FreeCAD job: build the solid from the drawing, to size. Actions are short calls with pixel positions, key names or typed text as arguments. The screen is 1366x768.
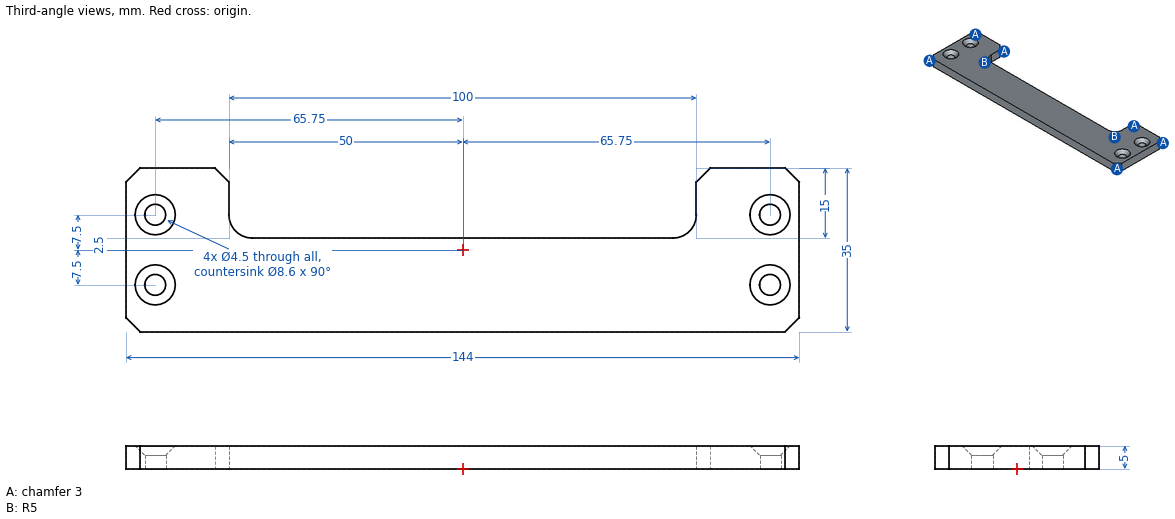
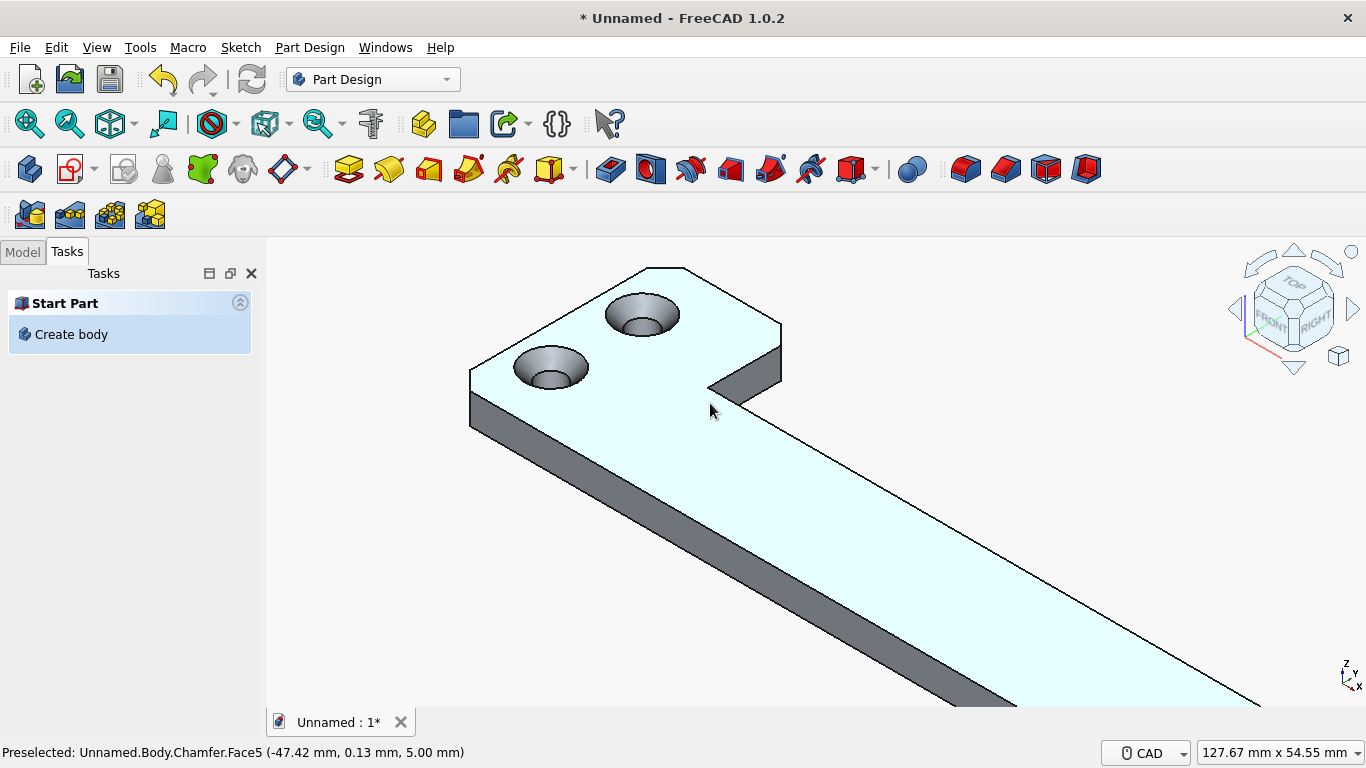
key(v)
key(f)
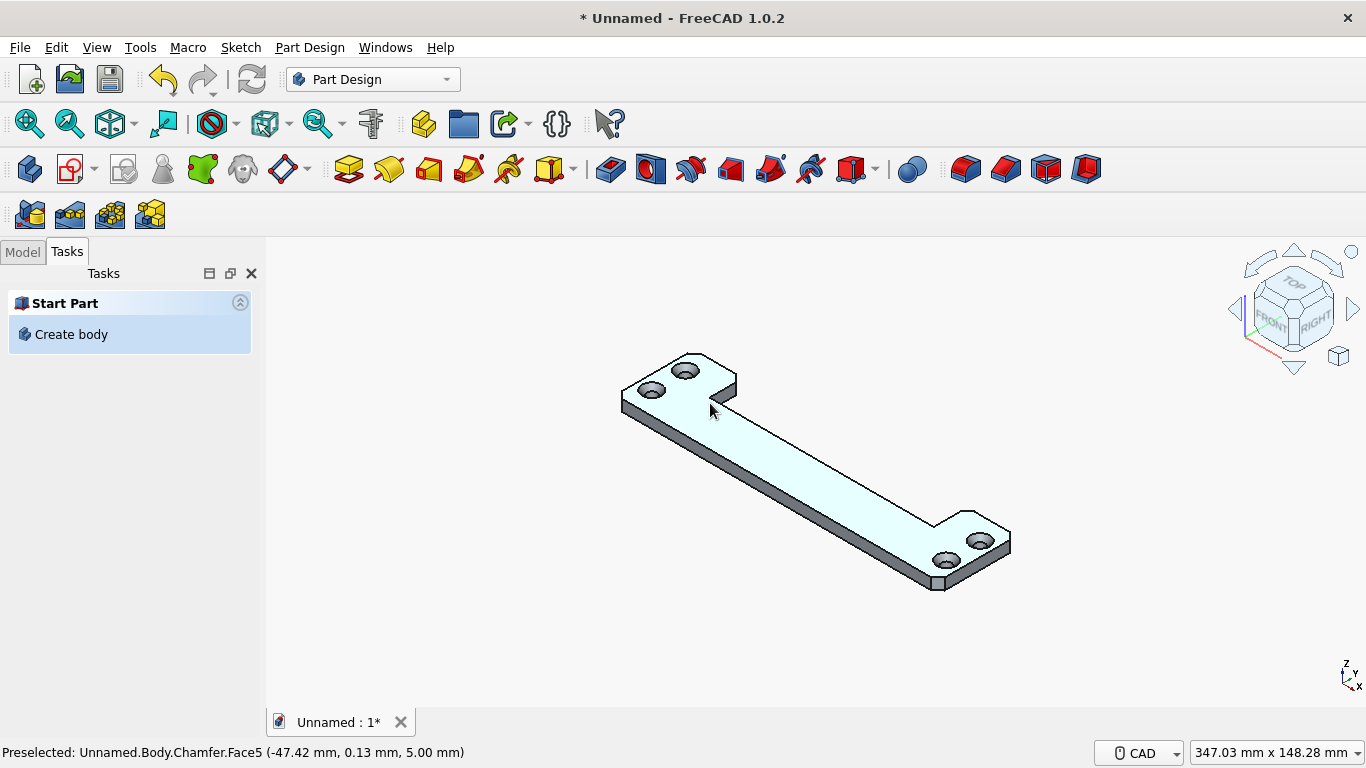
key(2)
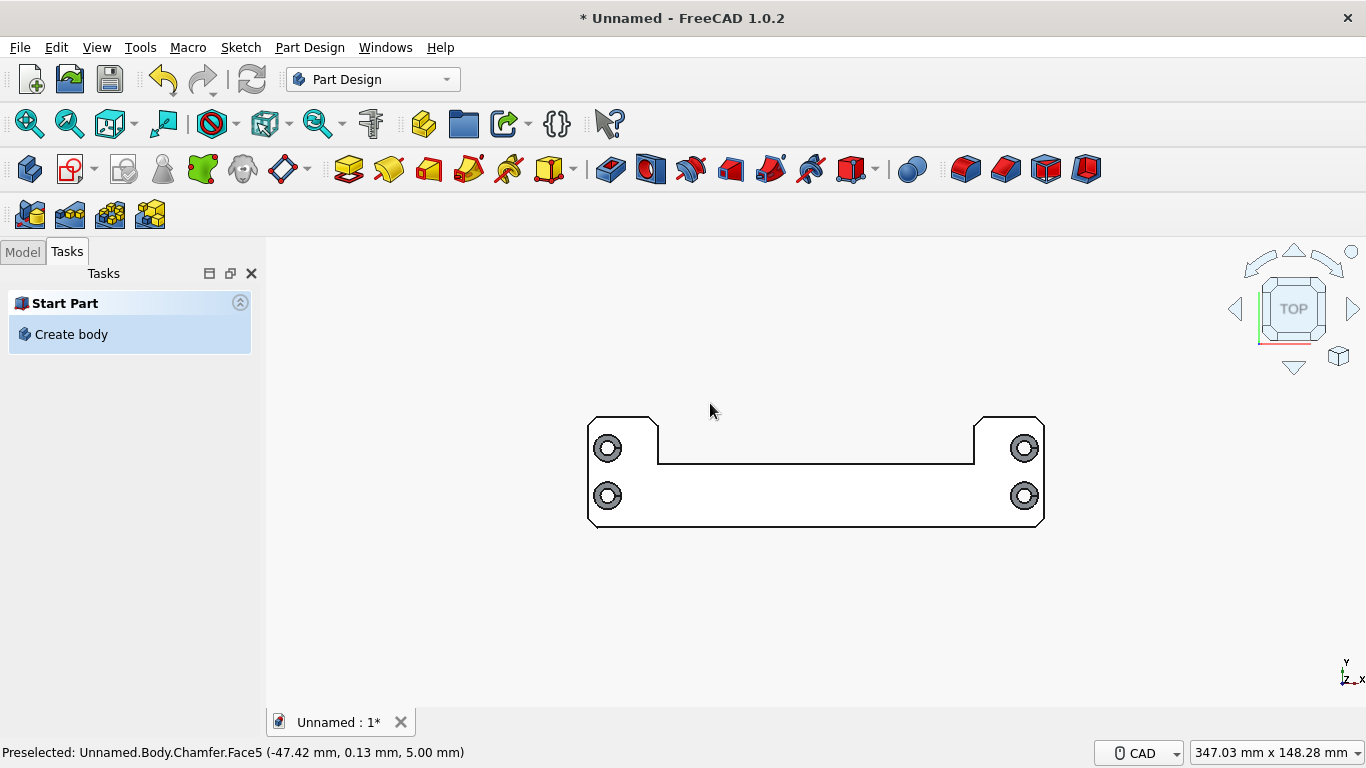
key(v)
key(f)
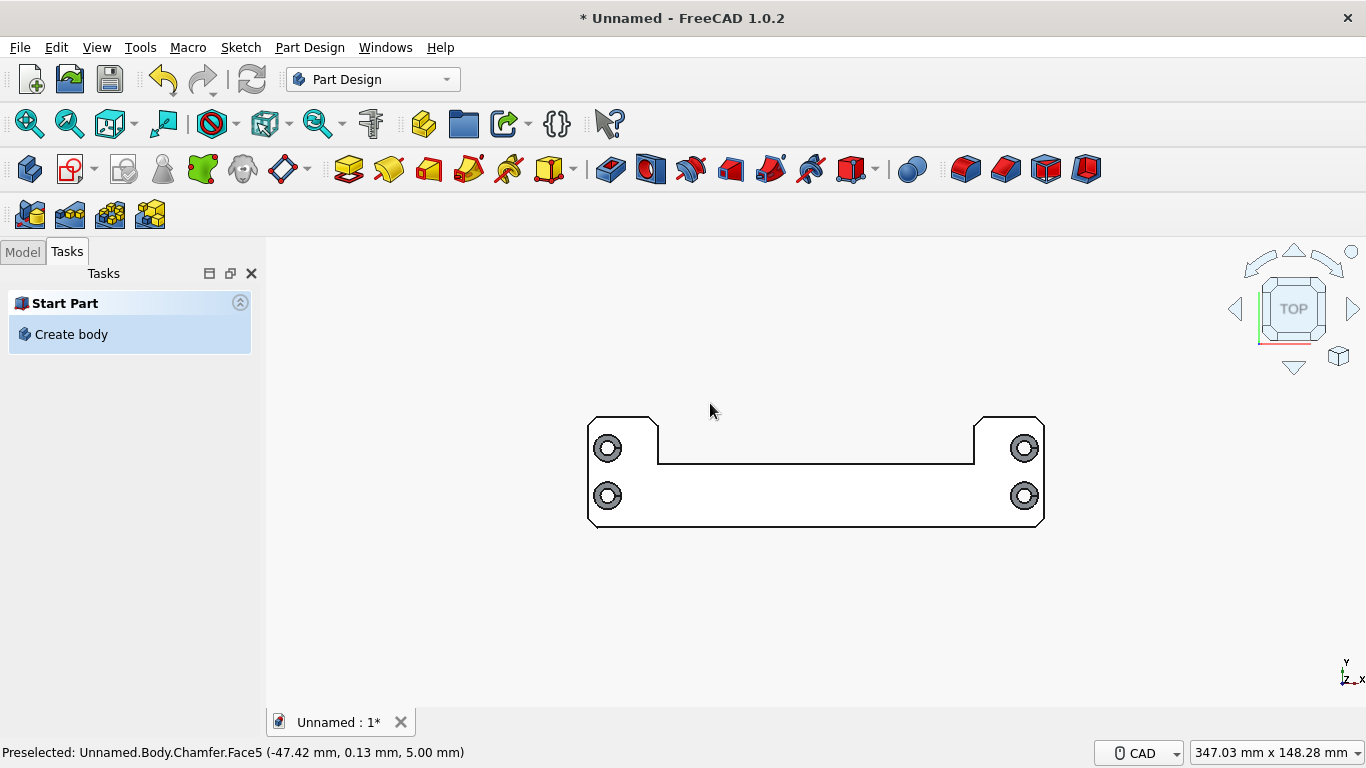
scroll(658, 463, up, 5)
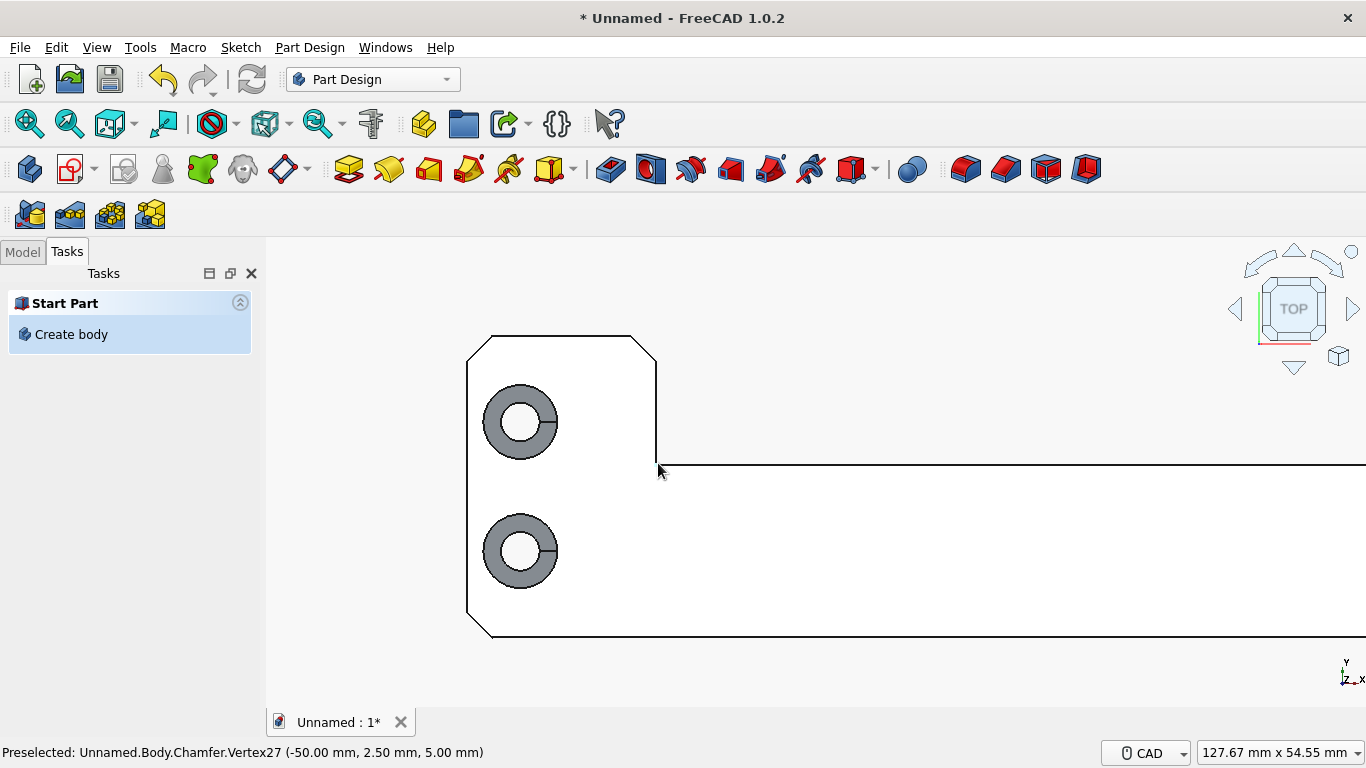
key(v)
key(f)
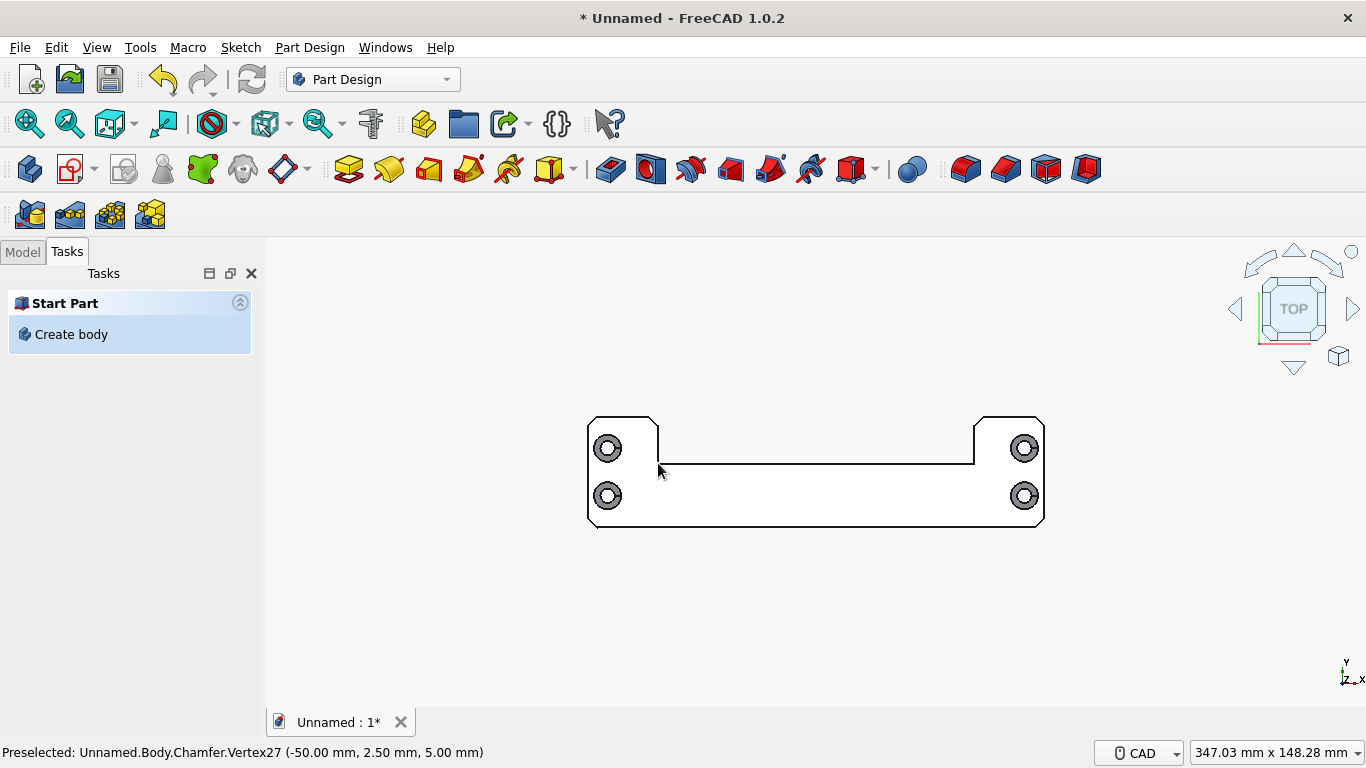
key(1)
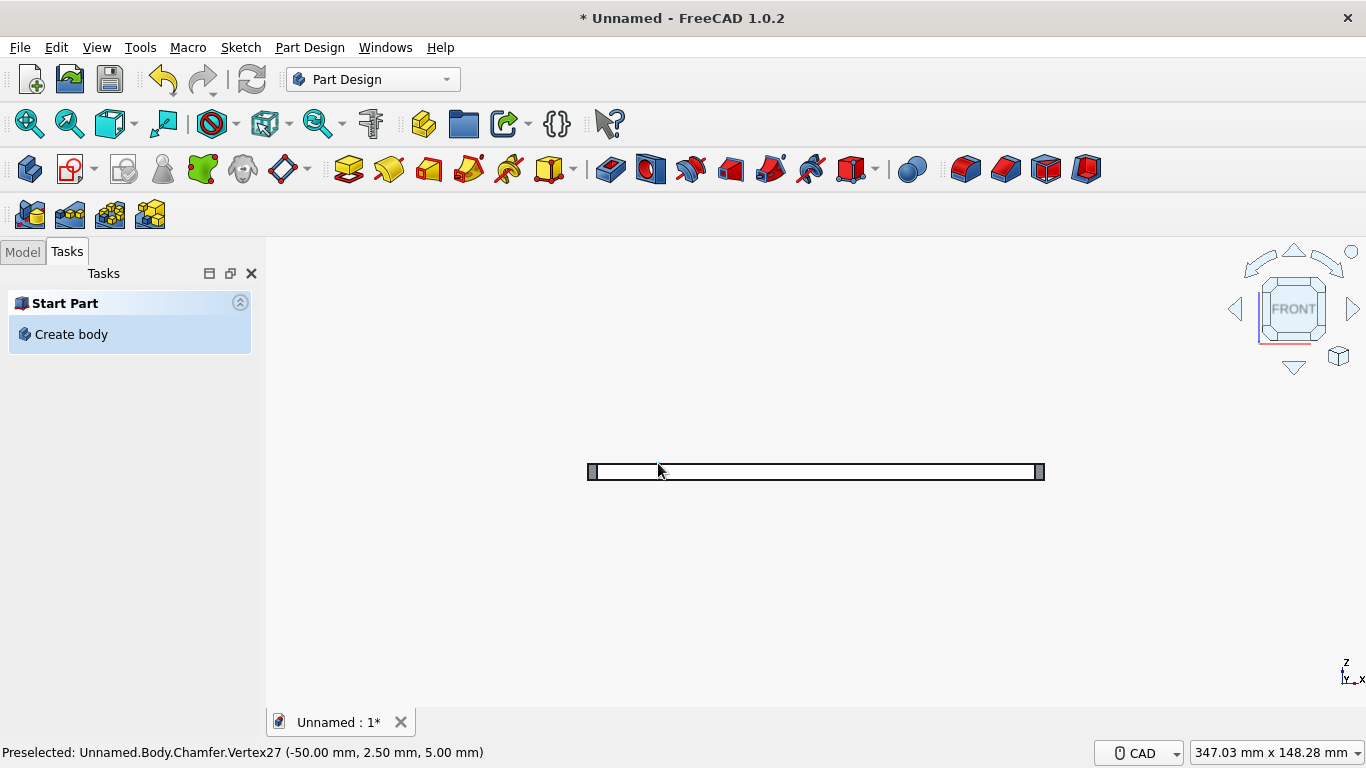
key(v)
key(f)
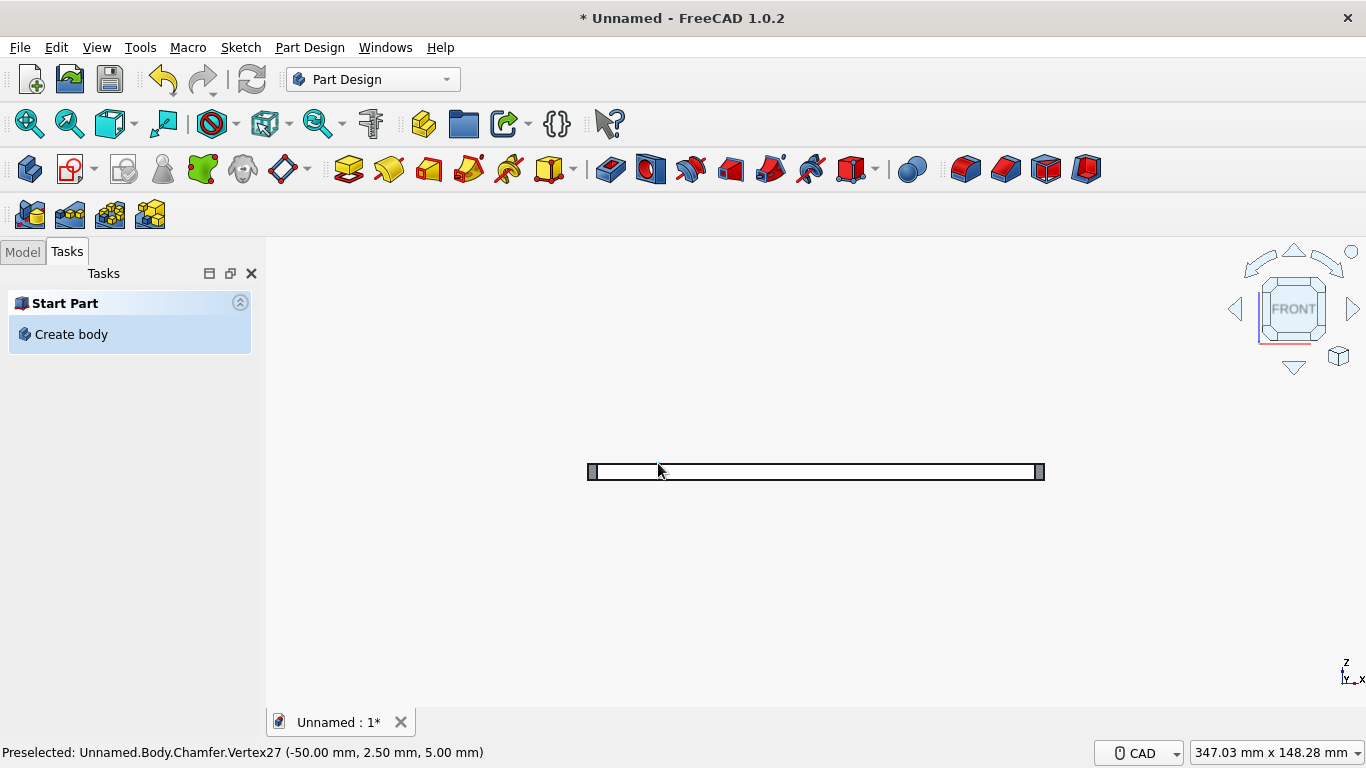
scroll(658, 471, up, 5)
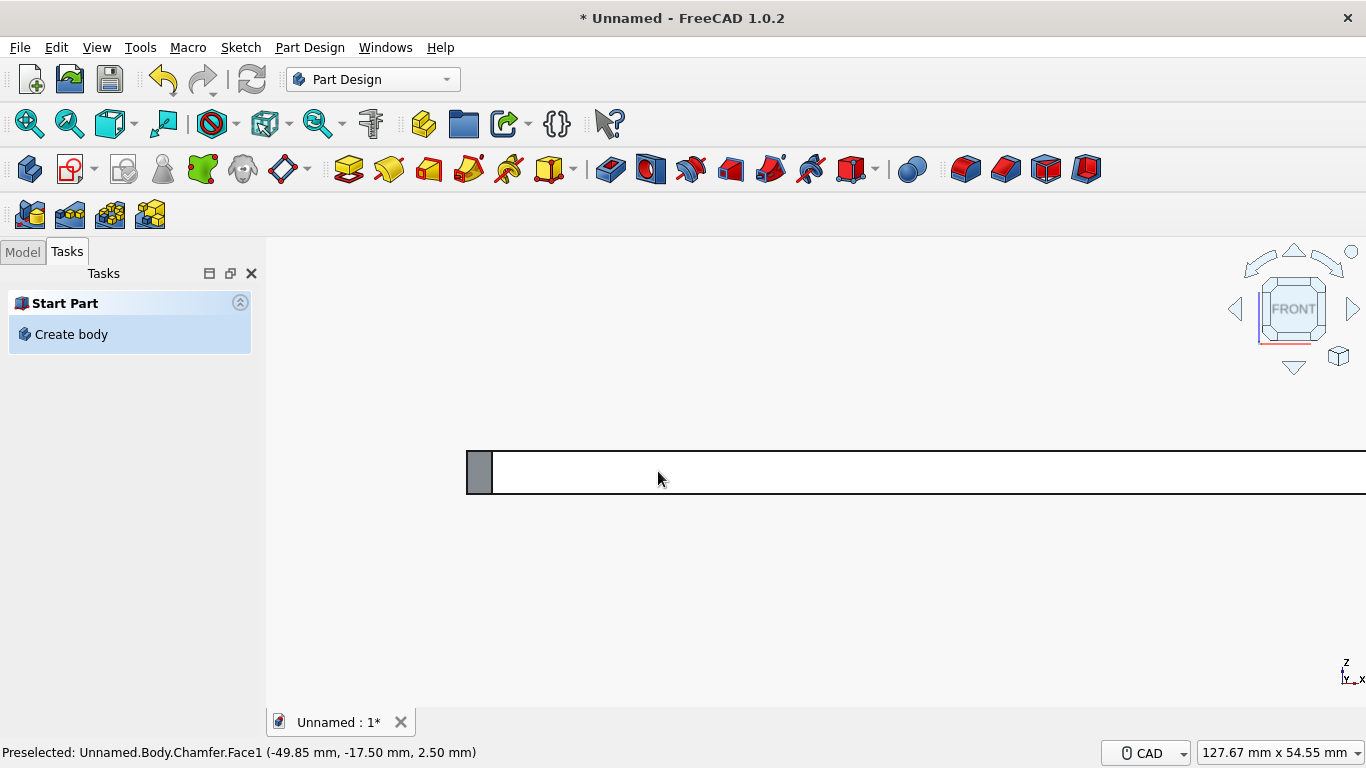
click(30, 124)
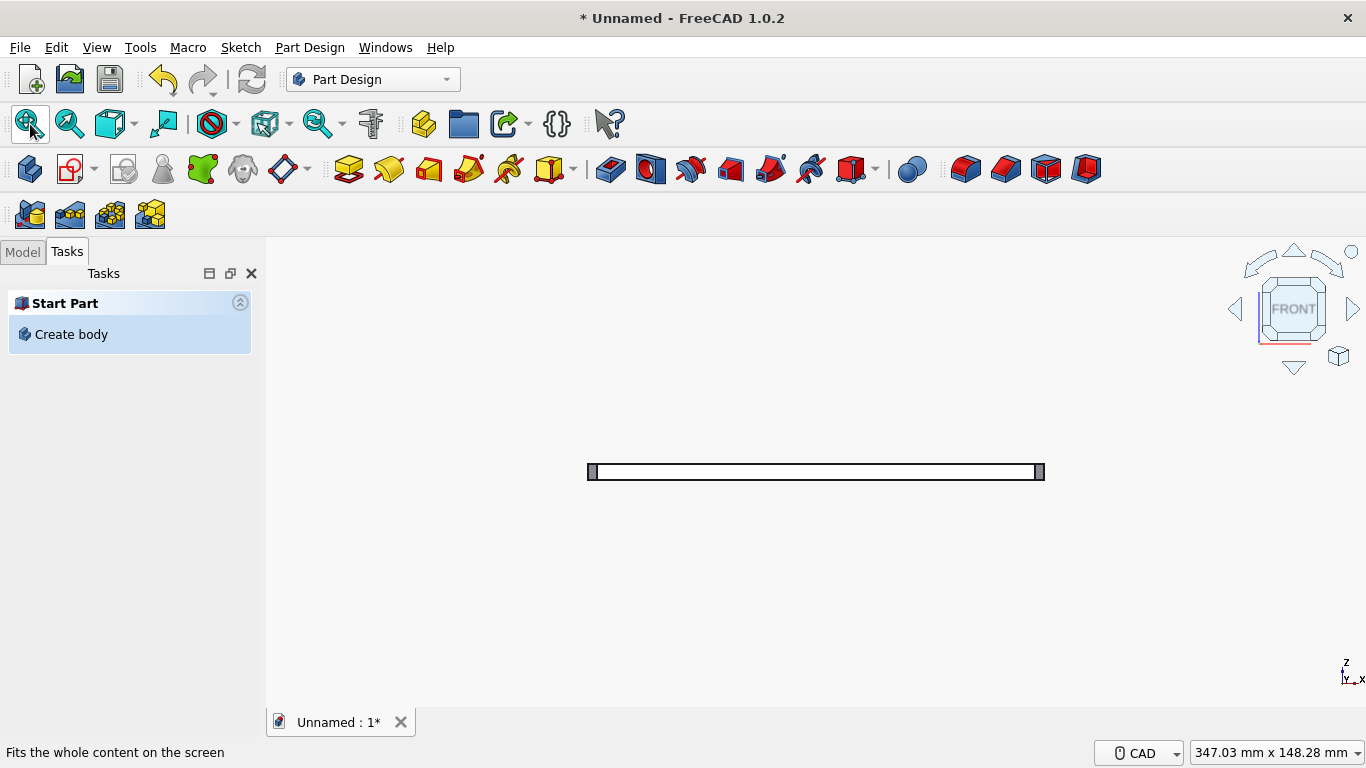
key(3)